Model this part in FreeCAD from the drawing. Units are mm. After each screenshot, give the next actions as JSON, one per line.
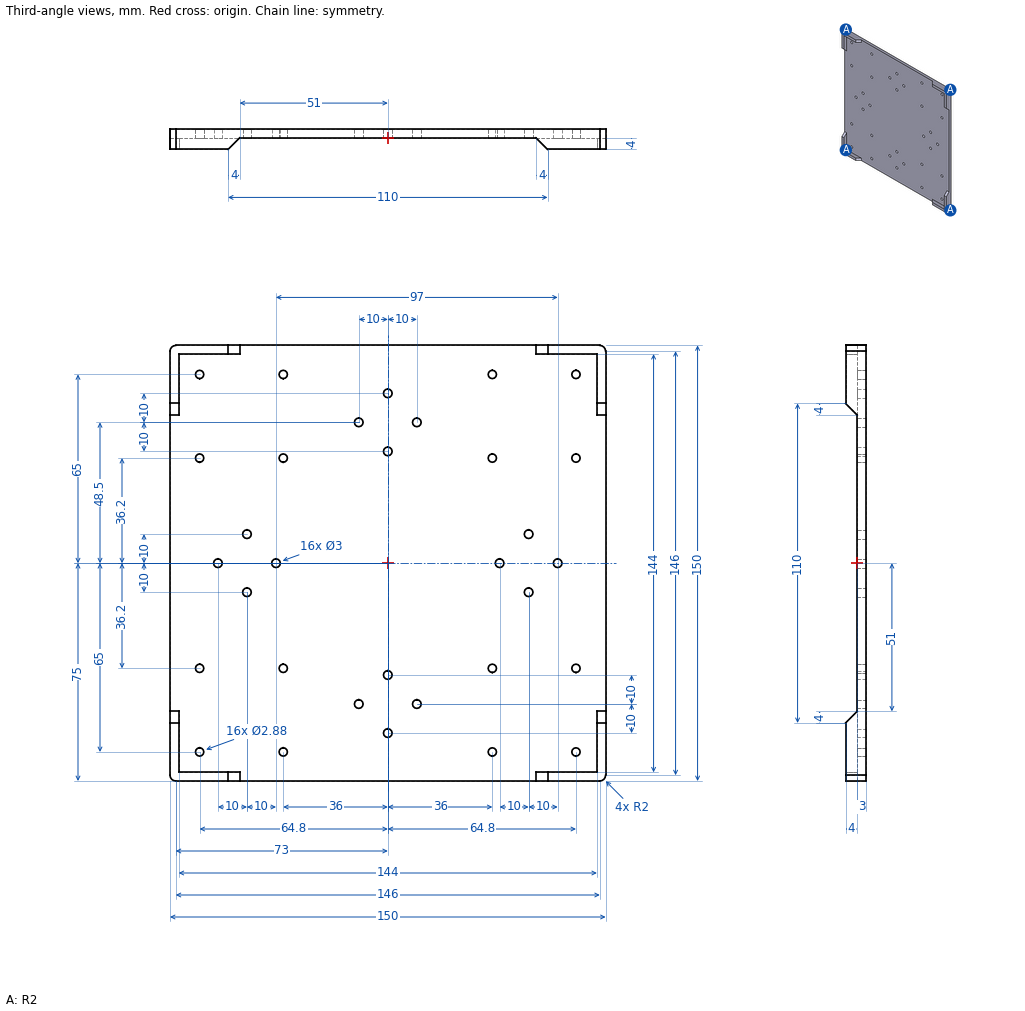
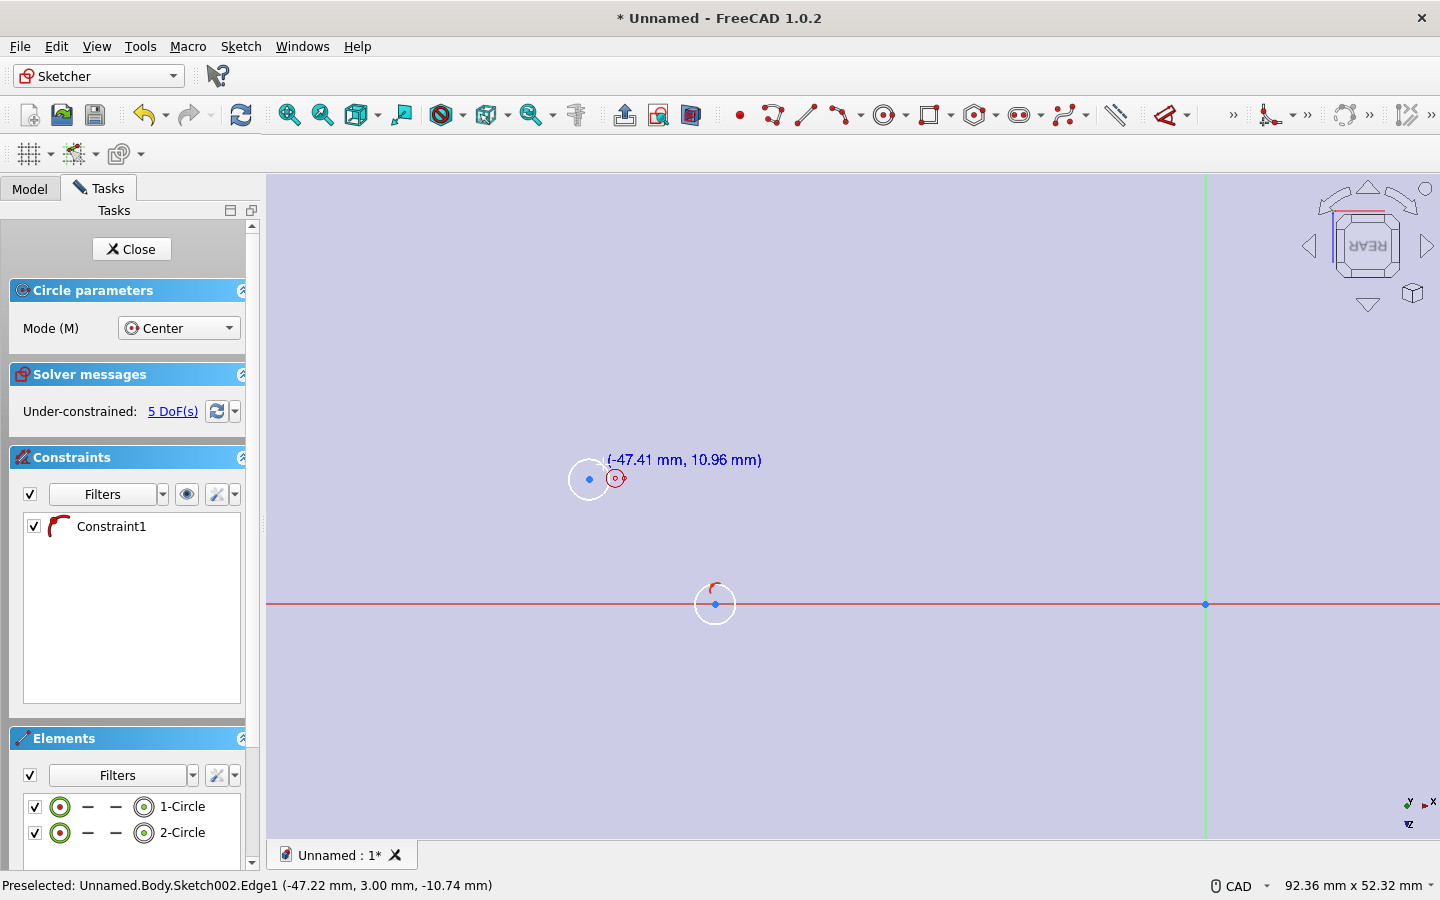
{"action": "scroll", "coordinate": [603, 464], "scroll_direction": "down", "scroll_amount": 6}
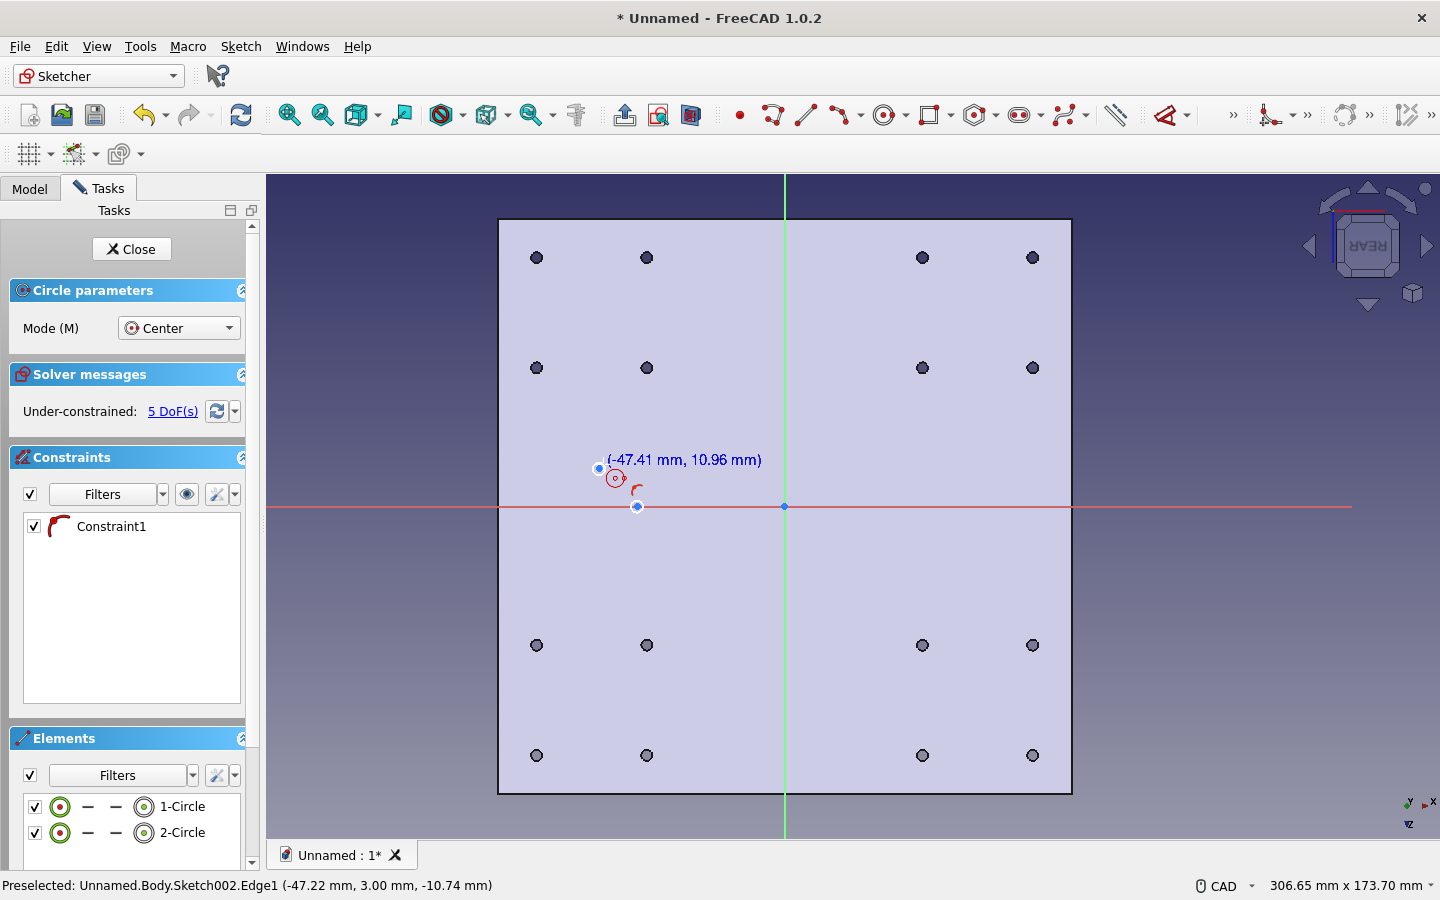
{"action": "left_click", "coordinate": [561, 507]}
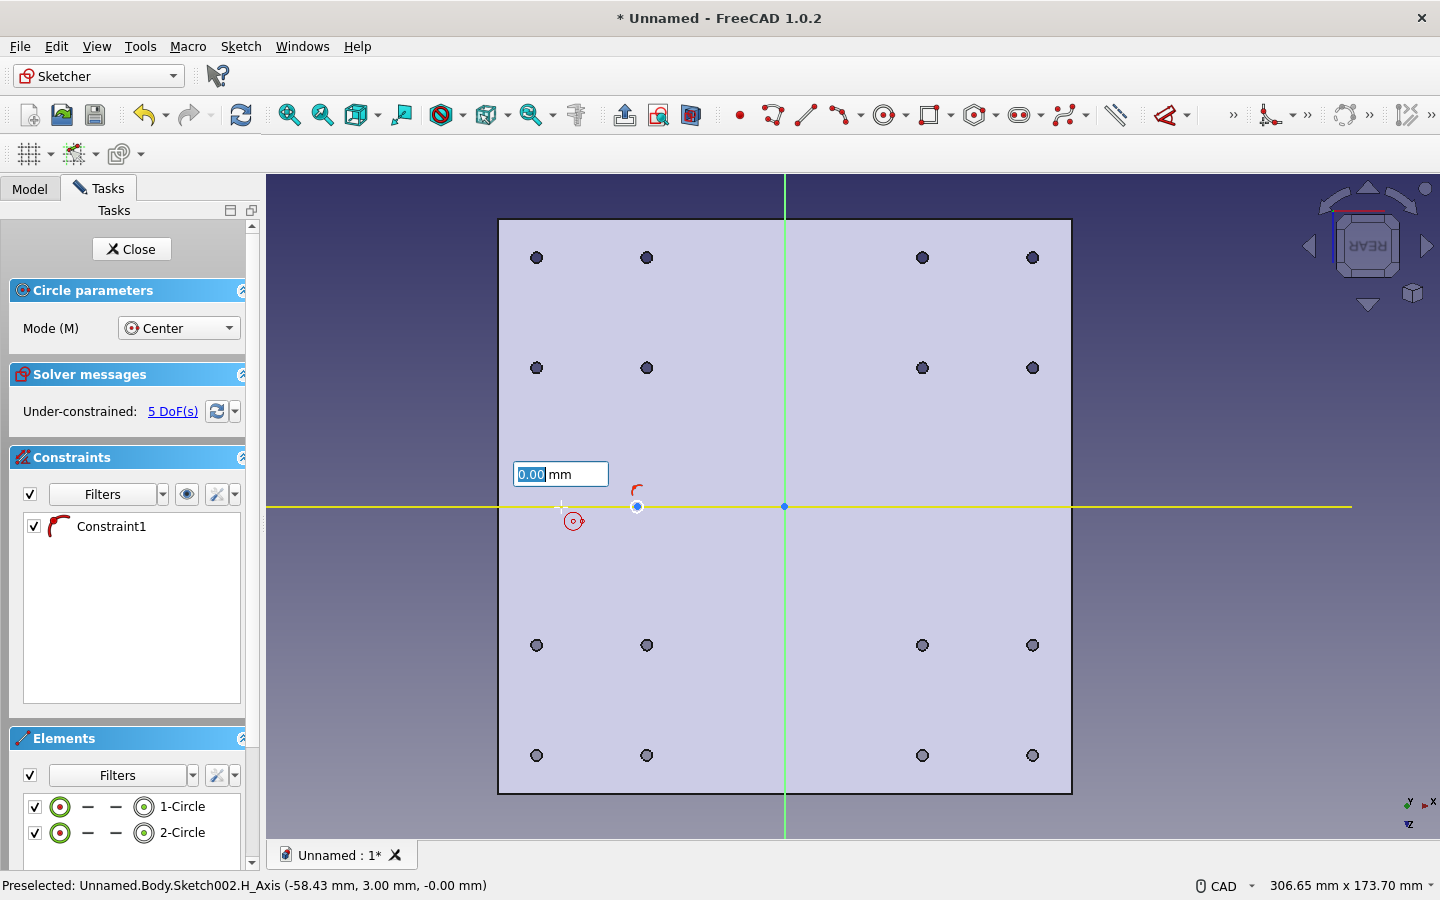
{"action": "scroll", "coordinate": [559, 512], "scroll_direction": "up", "scroll_amount": 6}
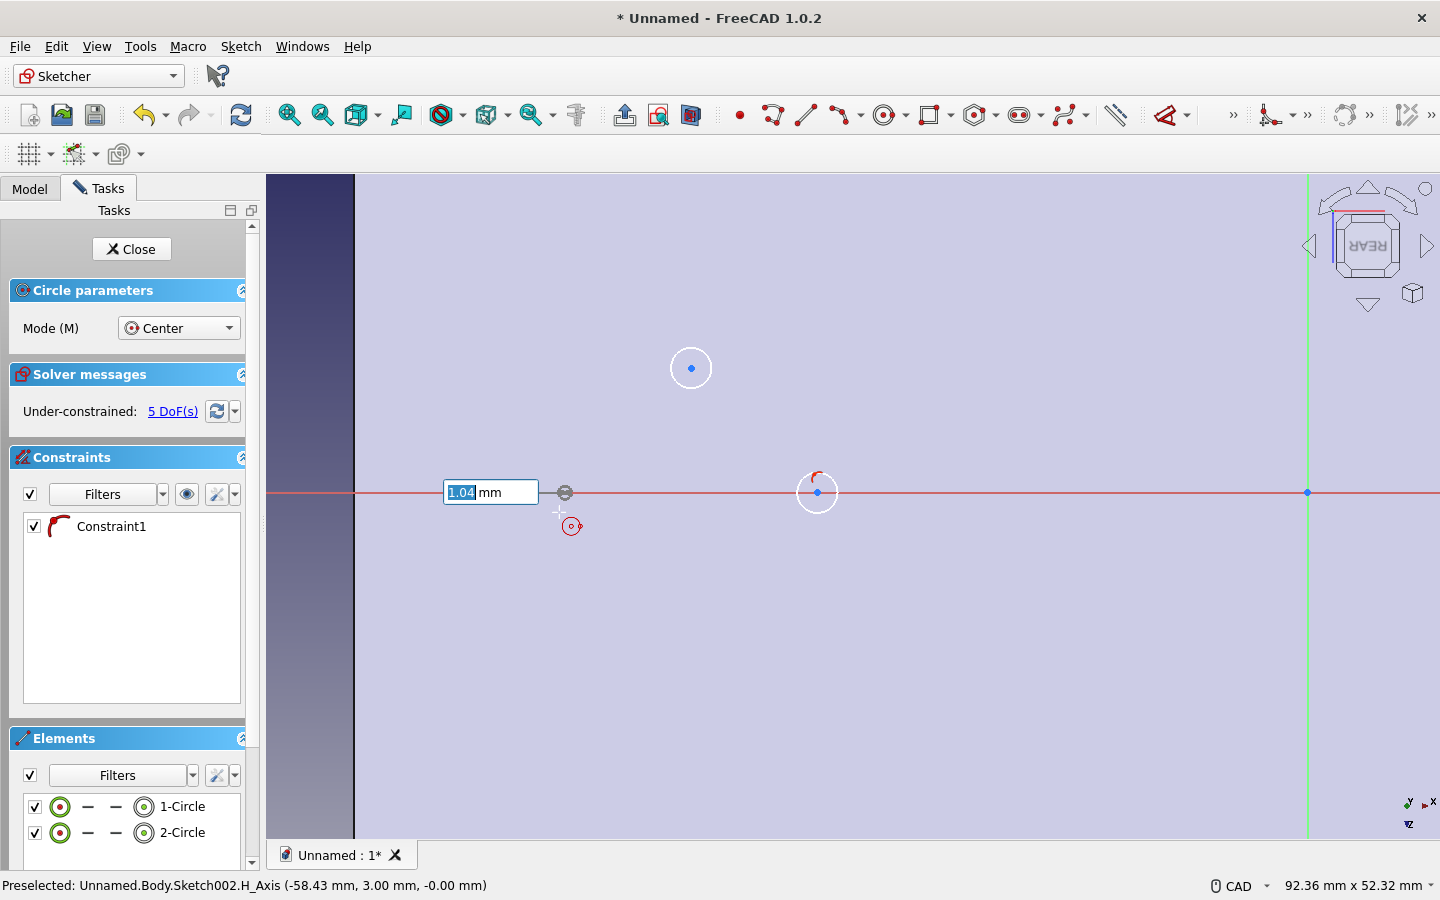
{"action": "left_click", "coordinate": [558, 511]}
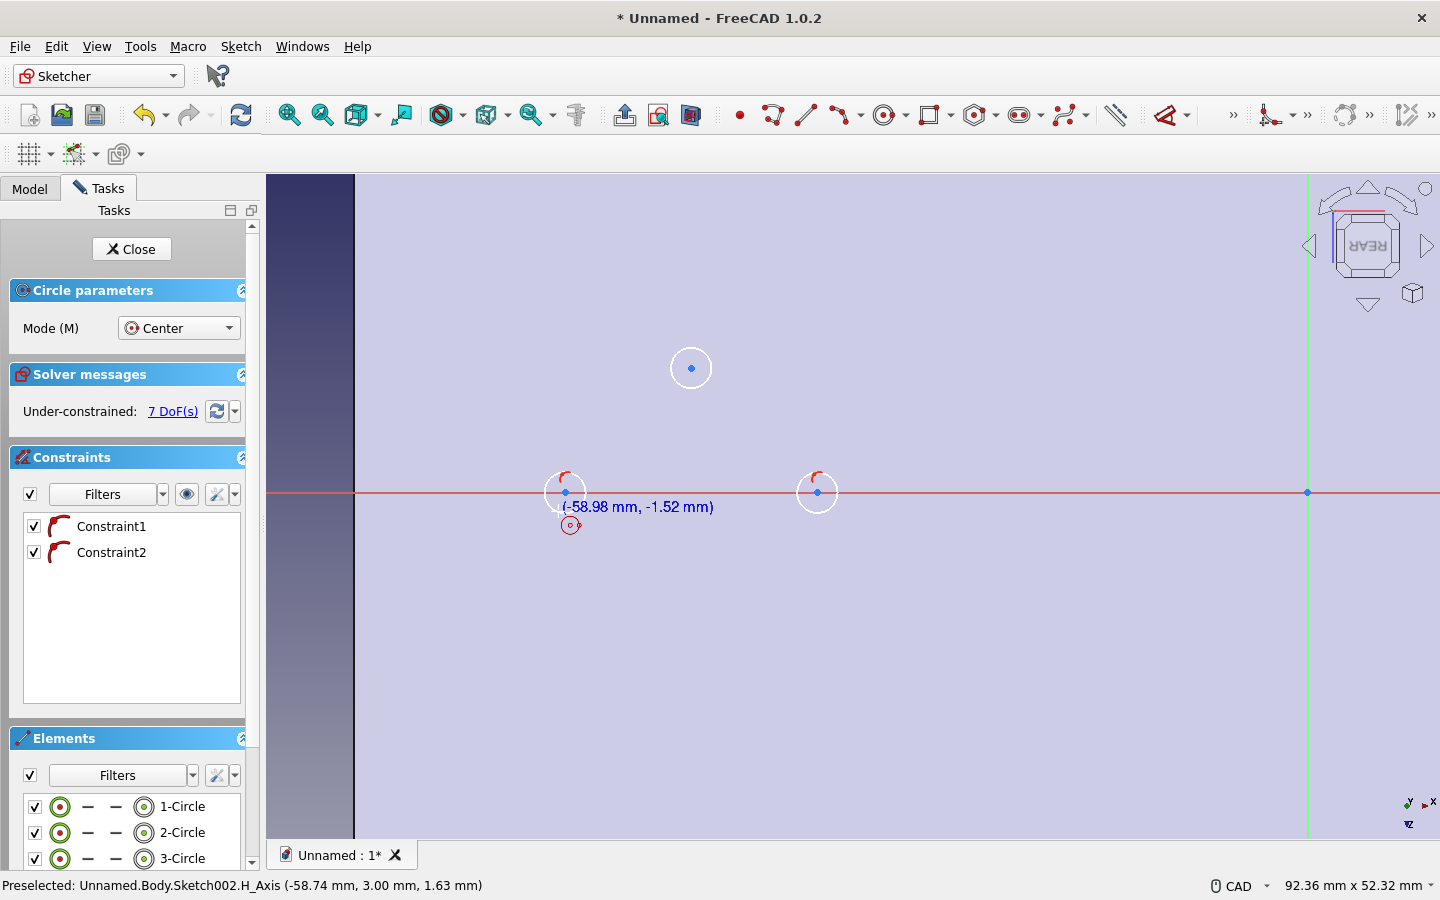
{"action": "scroll", "coordinate": [559, 512], "scroll_direction": "down", "scroll_amount": 6}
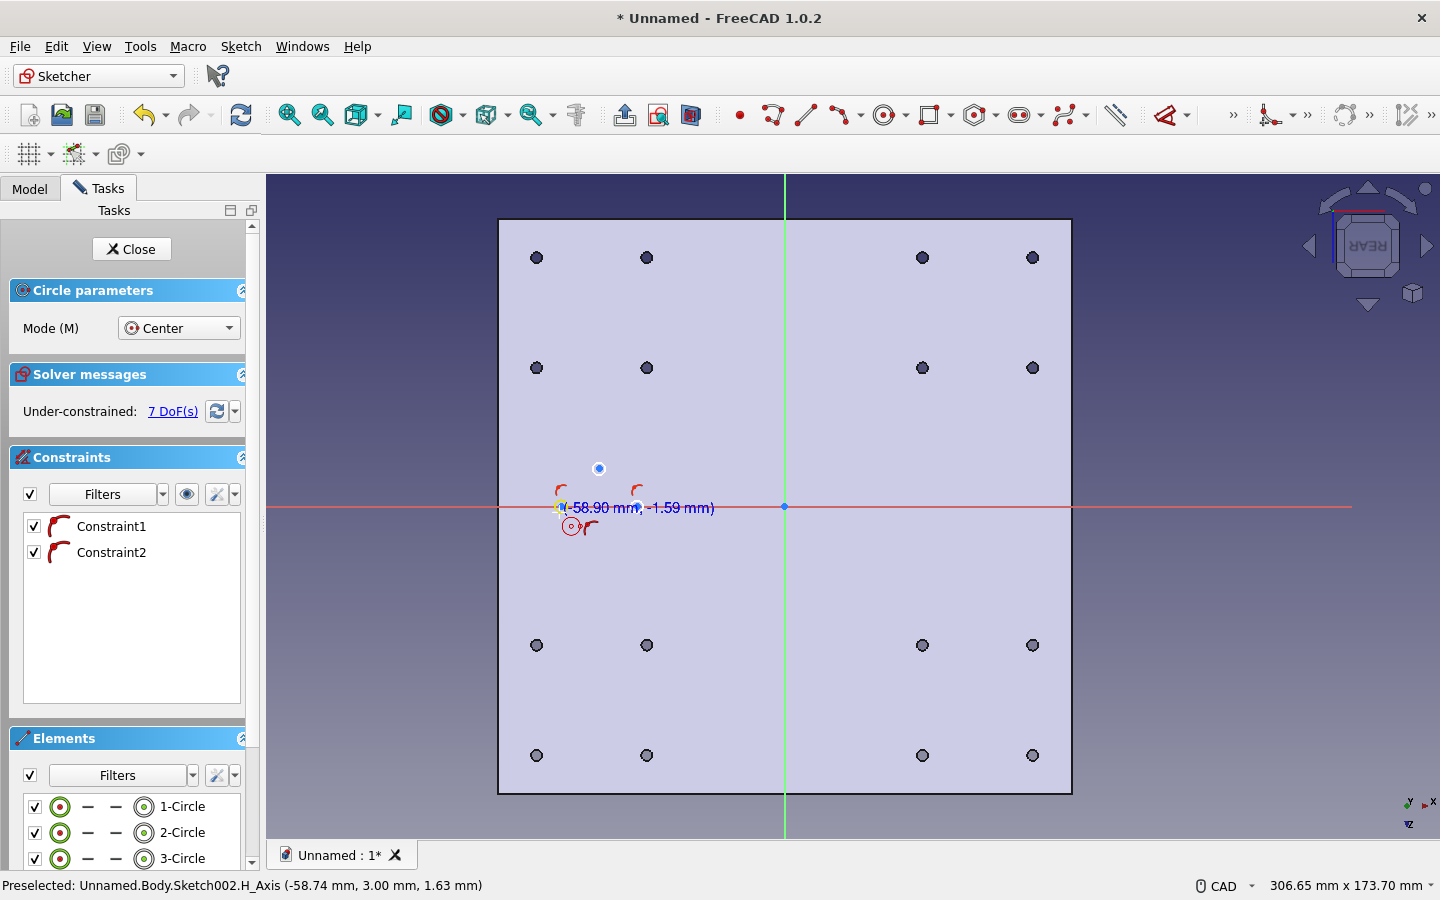
{"action": "left_click", "coordinate": [599, 545]}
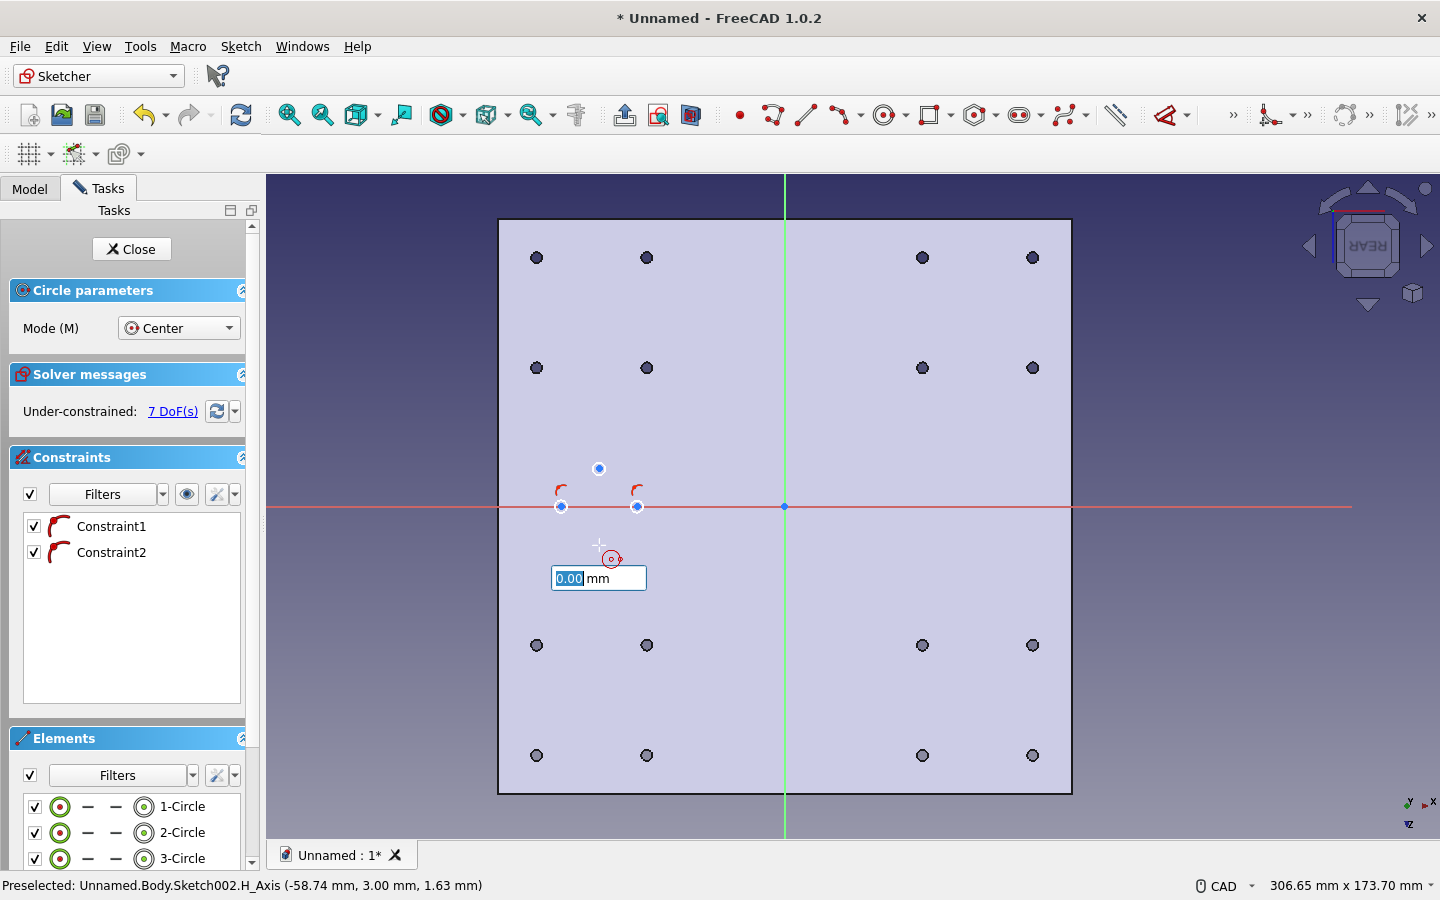
{"action": "scroll", "coordinate": [603, 541], "scroll_direction": "up", "scroll_amount": 6}